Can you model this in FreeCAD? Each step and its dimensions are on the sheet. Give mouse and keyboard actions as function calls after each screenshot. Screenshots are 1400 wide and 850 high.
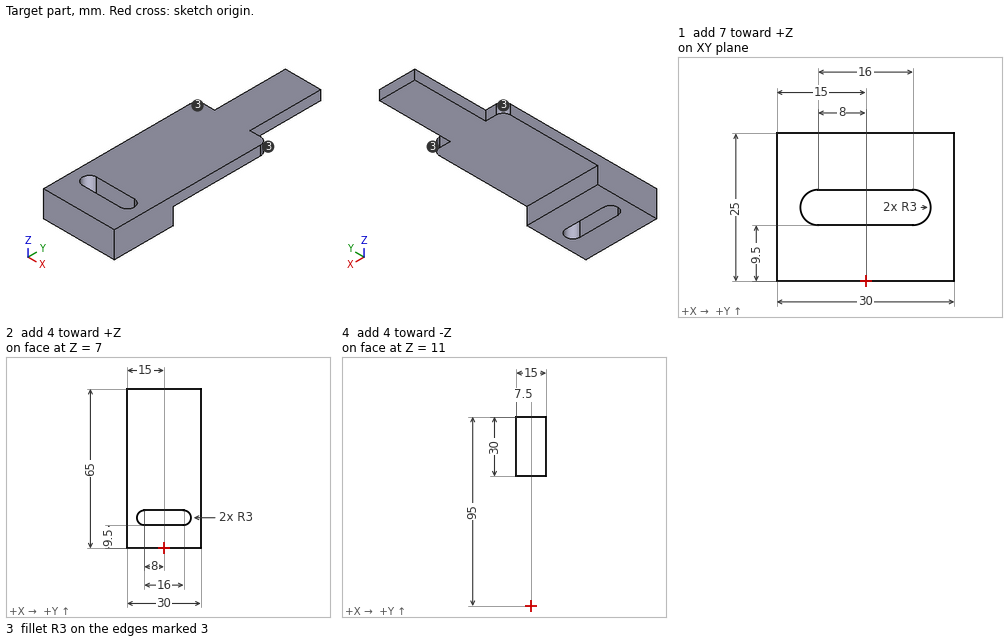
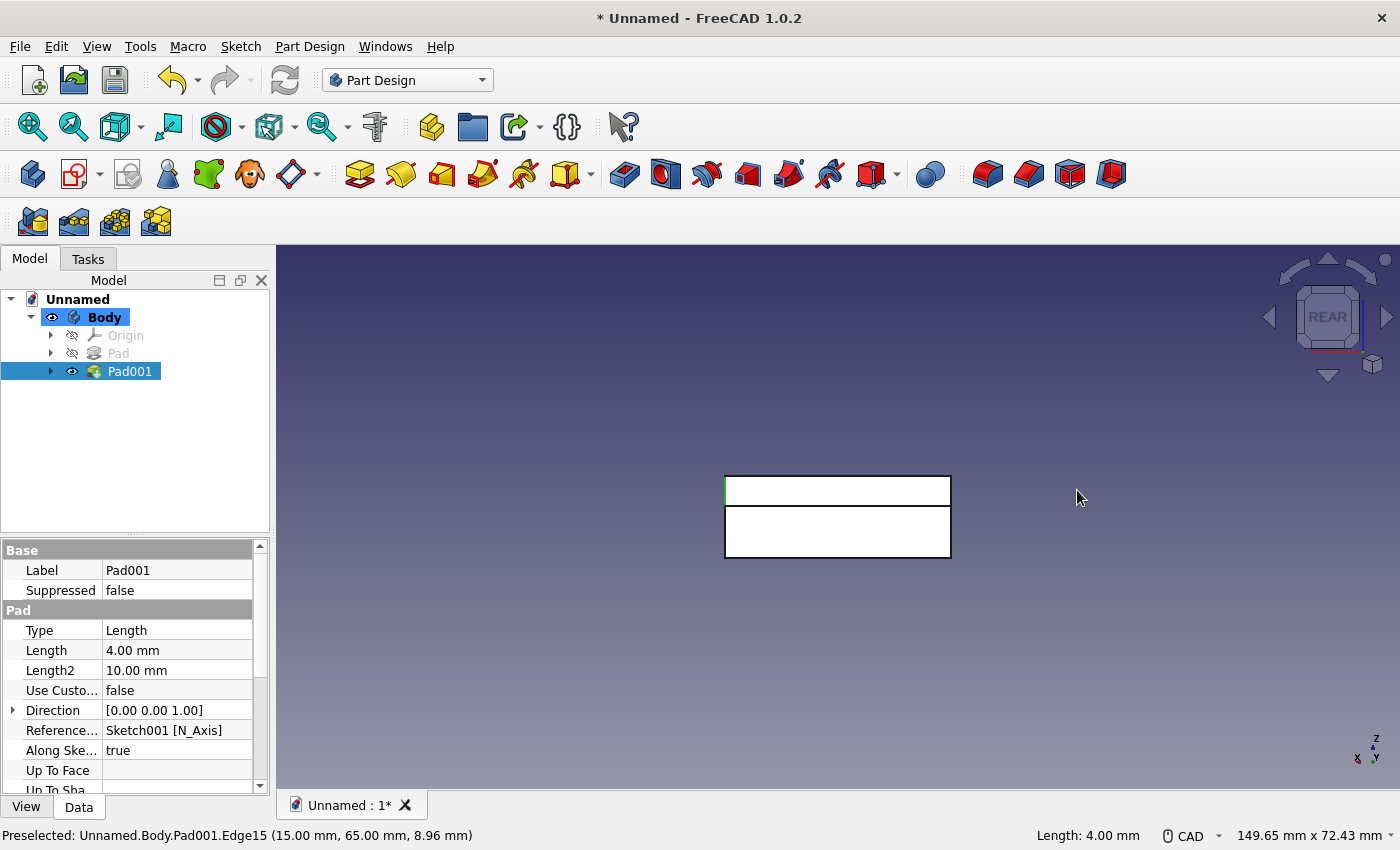
click(33, 128)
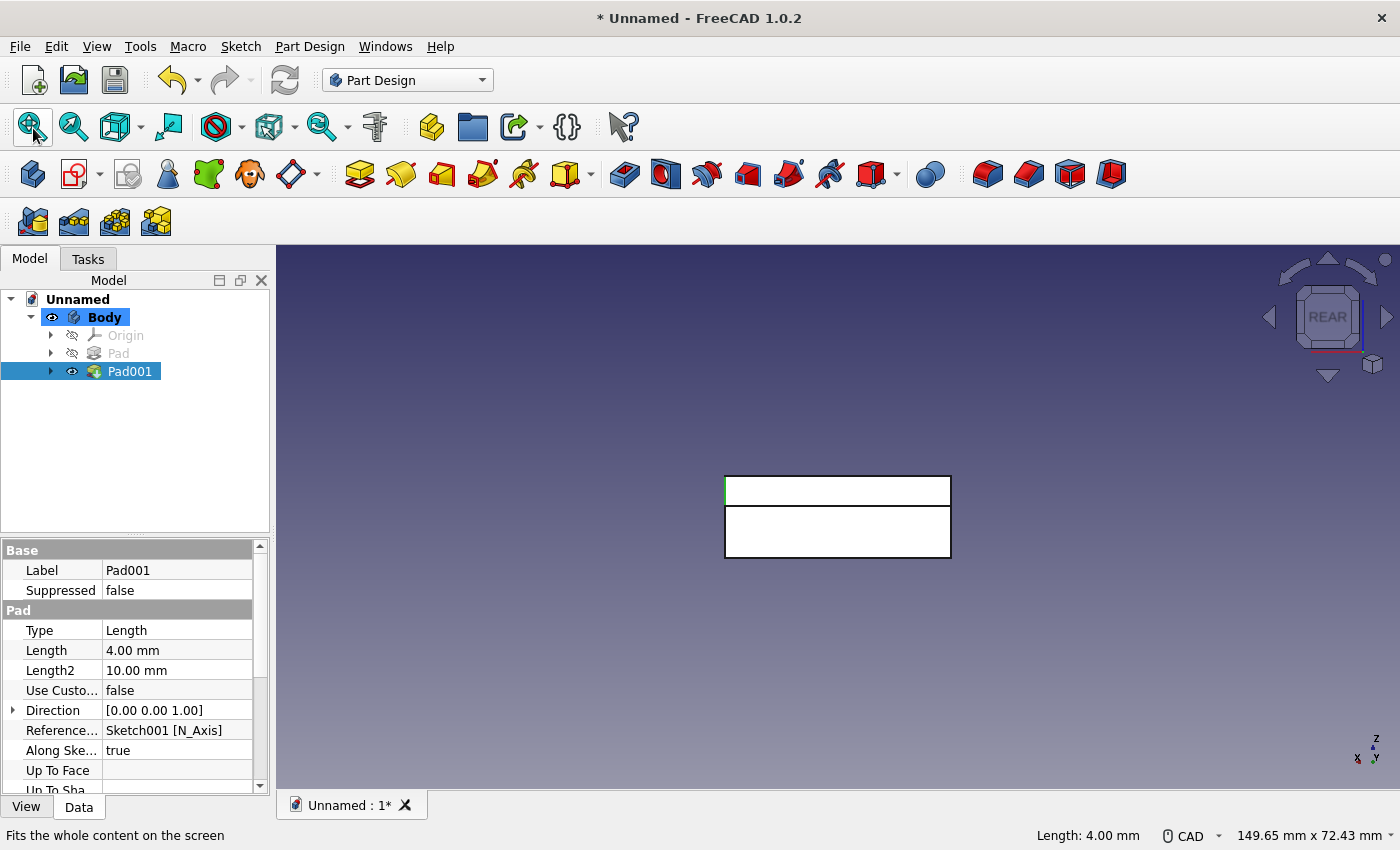
click(951, 490, ctrl)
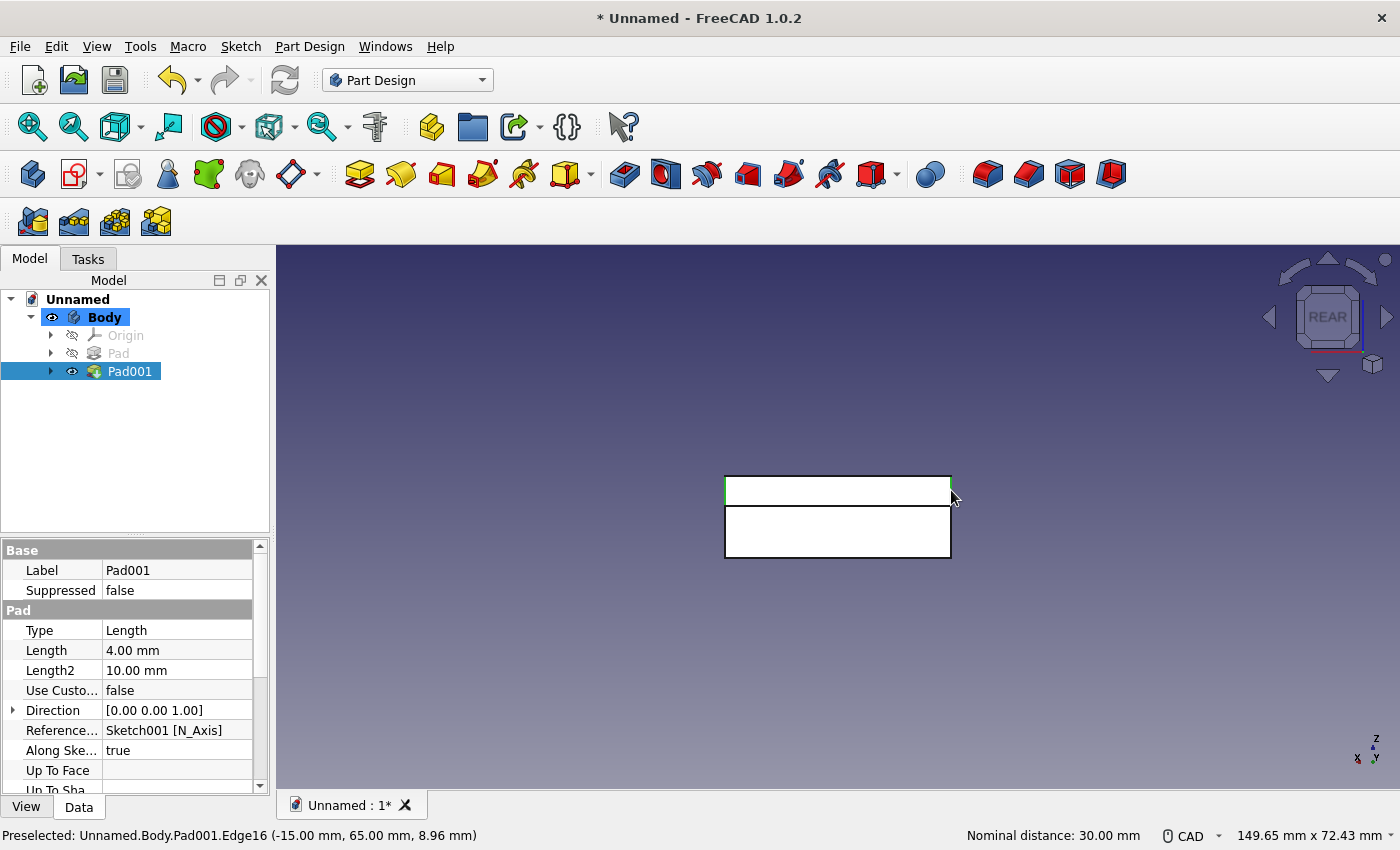
click(988, 174)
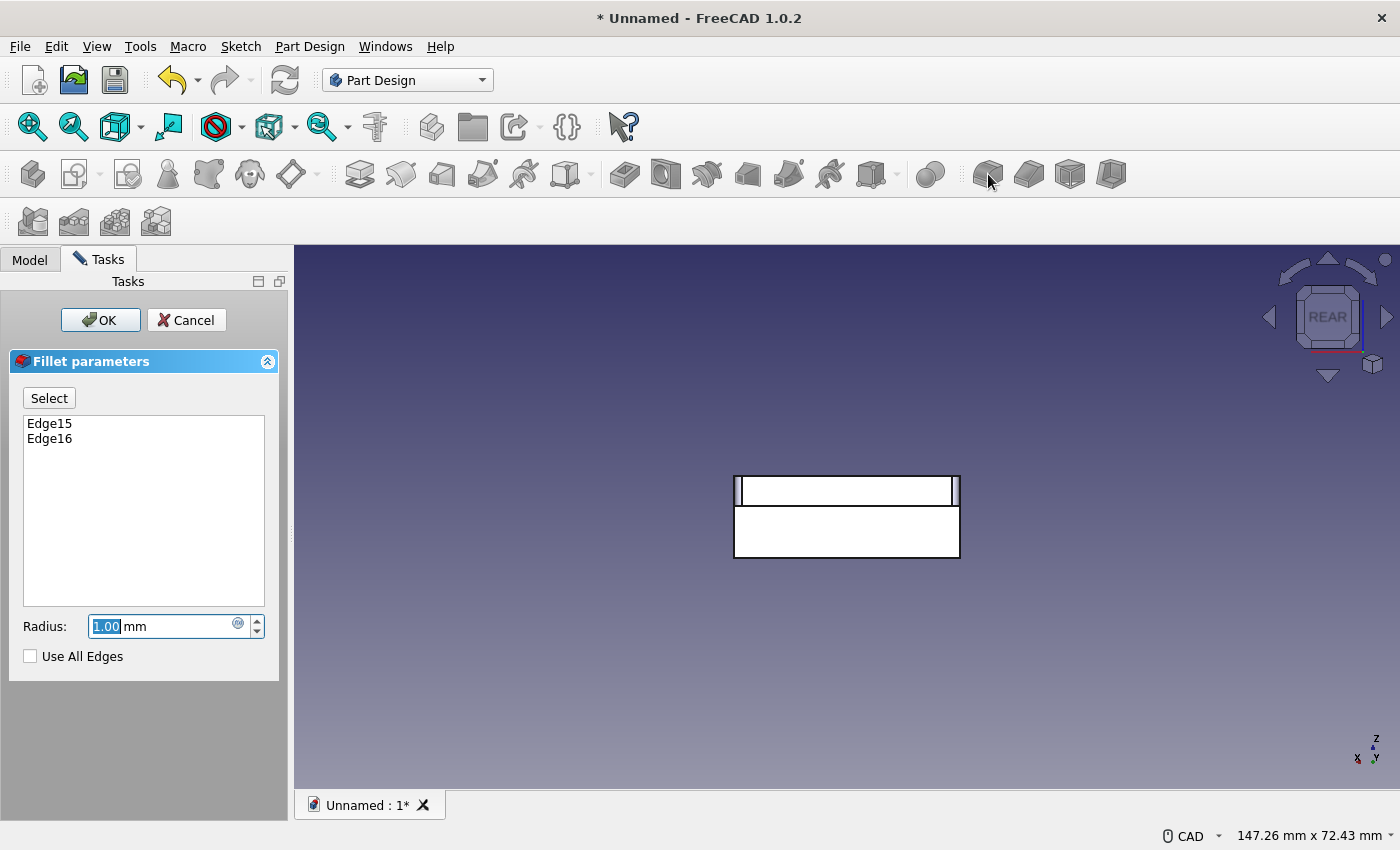
text(3)
key(Tab)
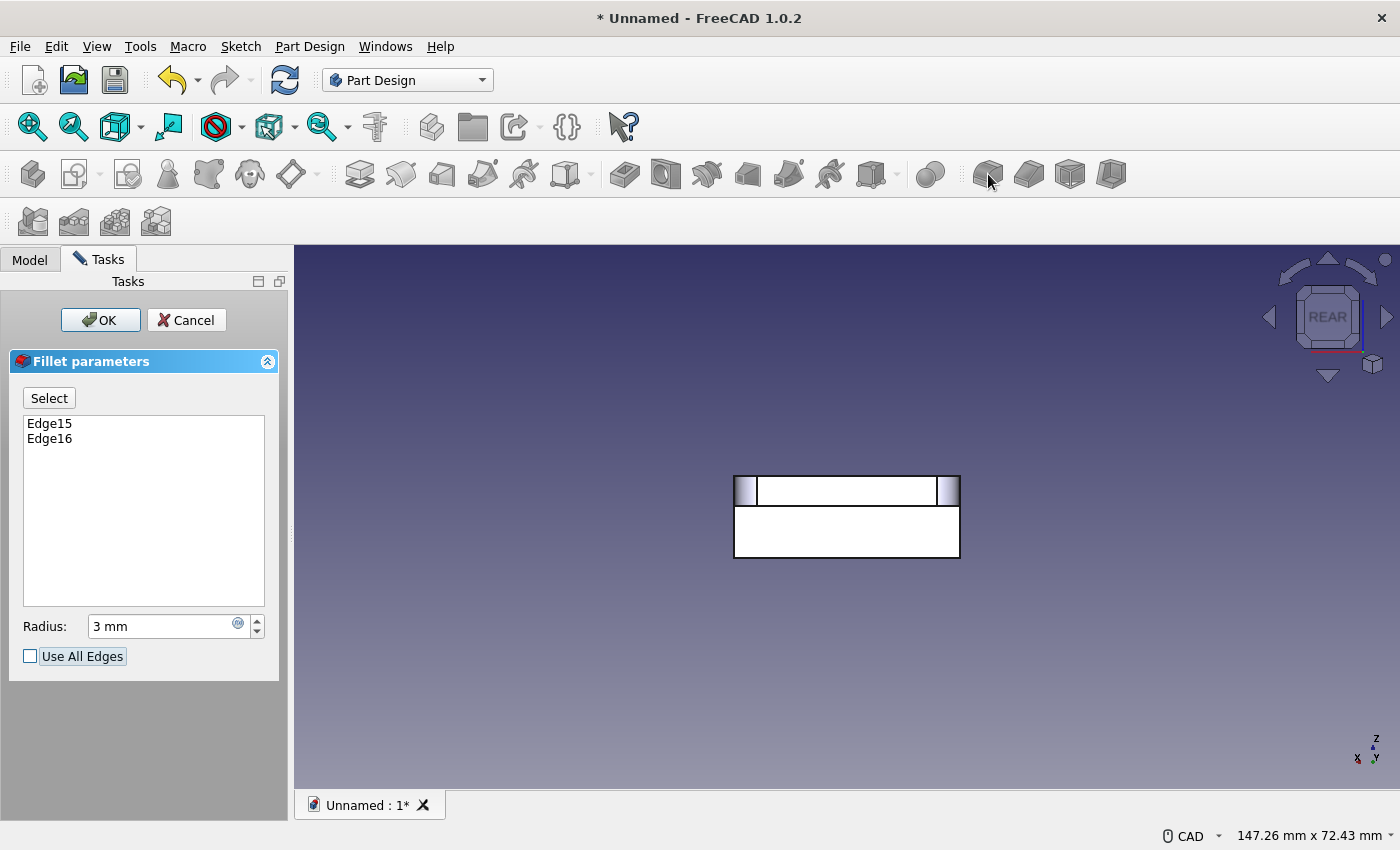
click(101, 320)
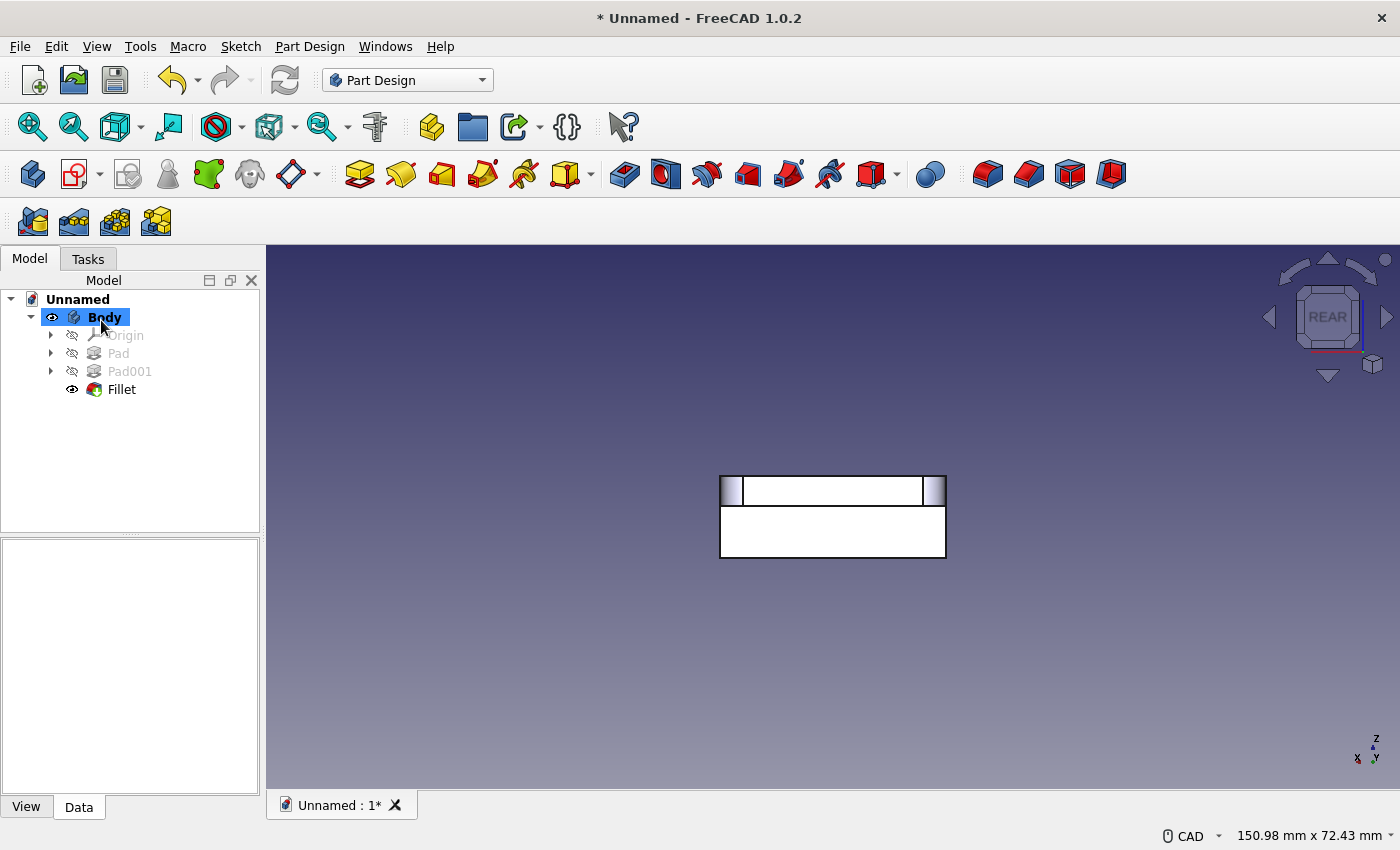
click(33, 128)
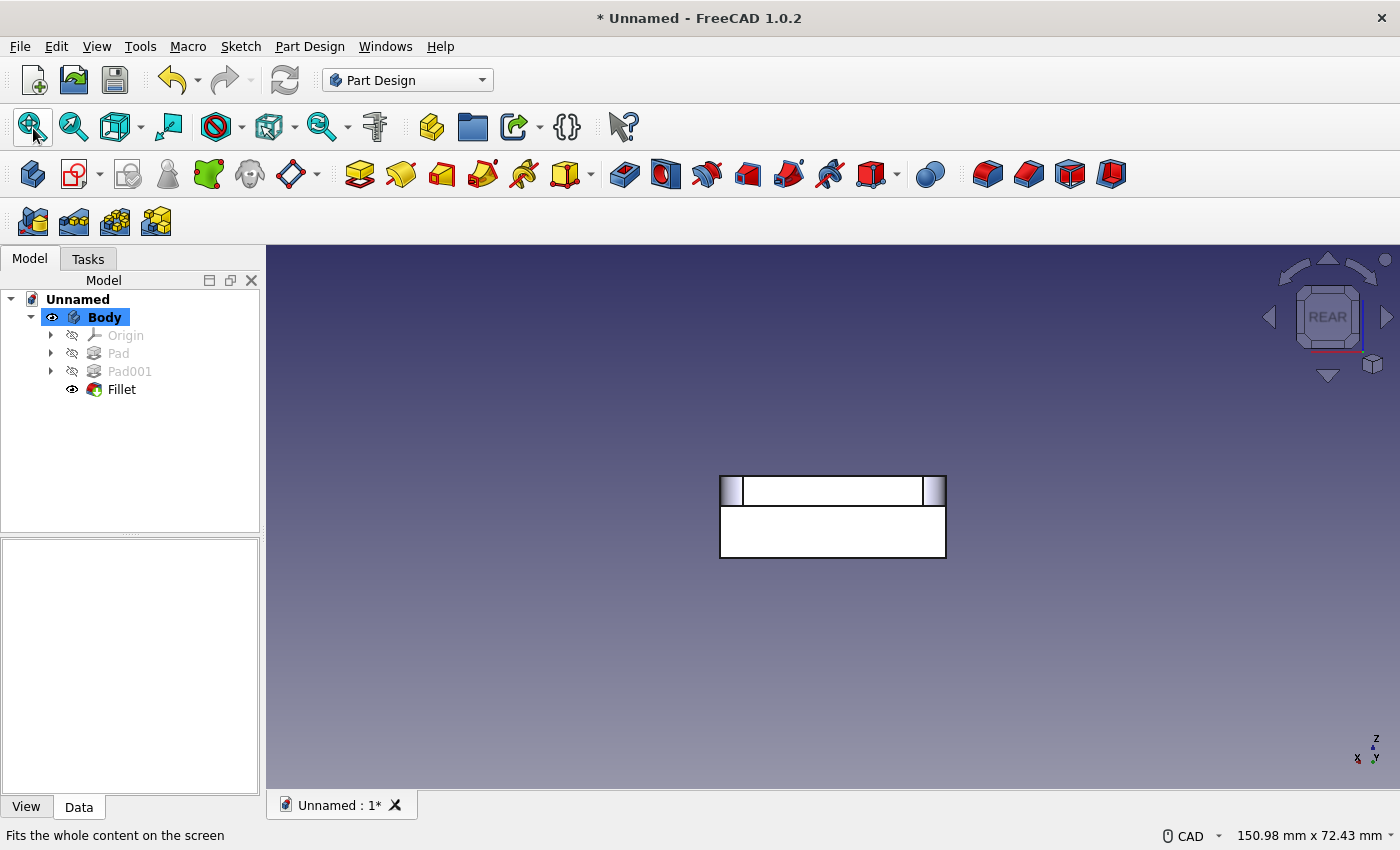
key(0)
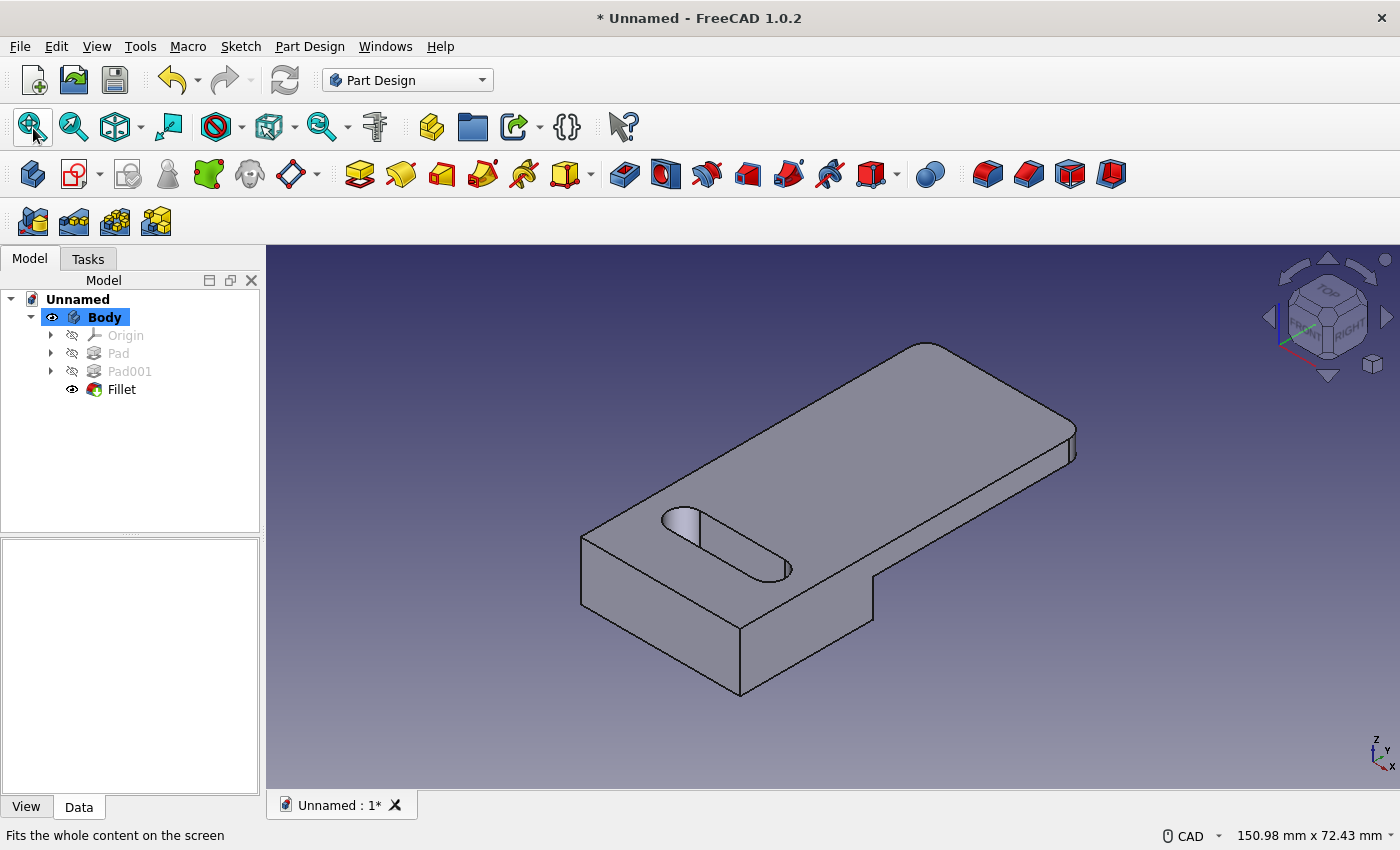
click(882, 454)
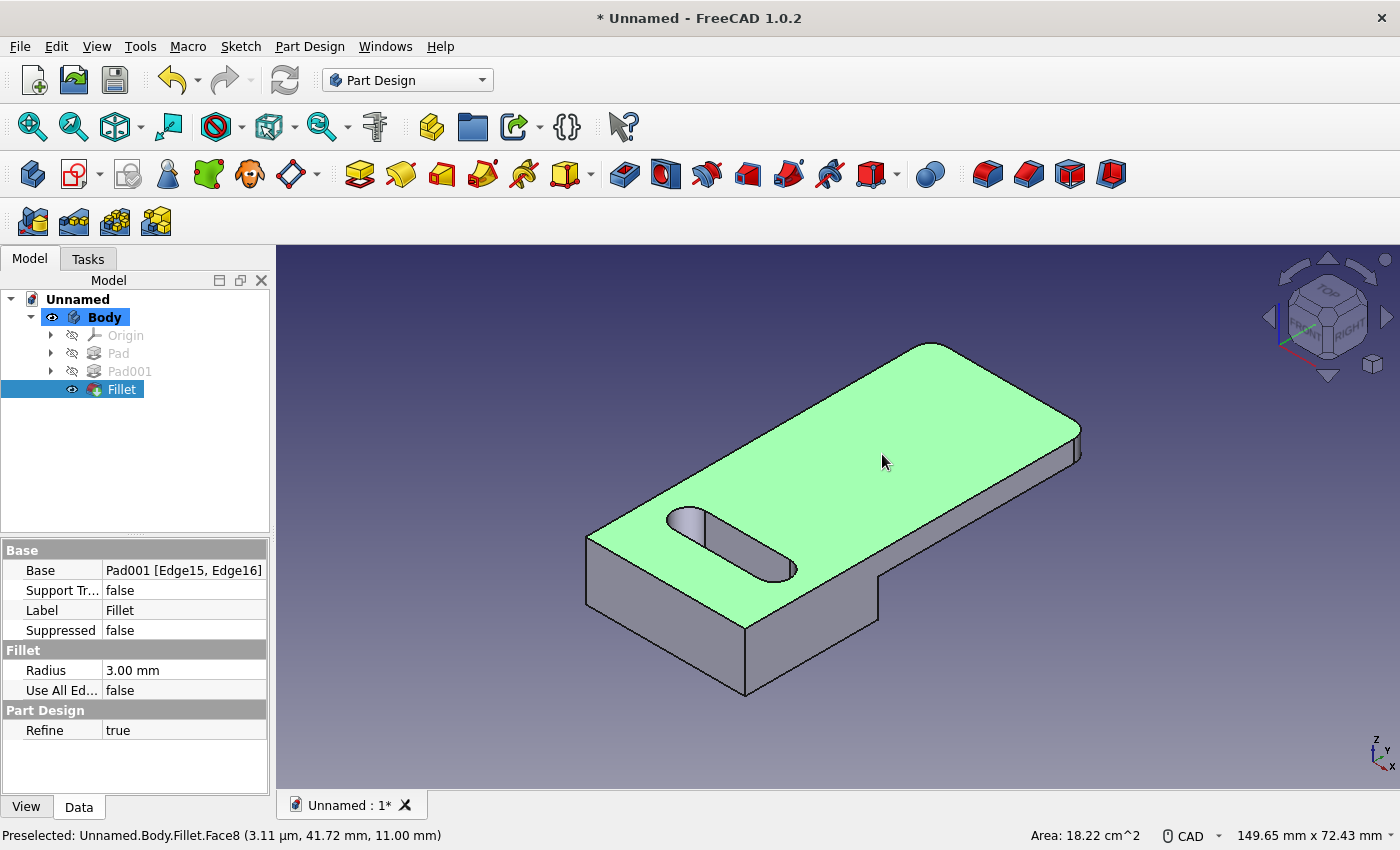
click(74, 174)